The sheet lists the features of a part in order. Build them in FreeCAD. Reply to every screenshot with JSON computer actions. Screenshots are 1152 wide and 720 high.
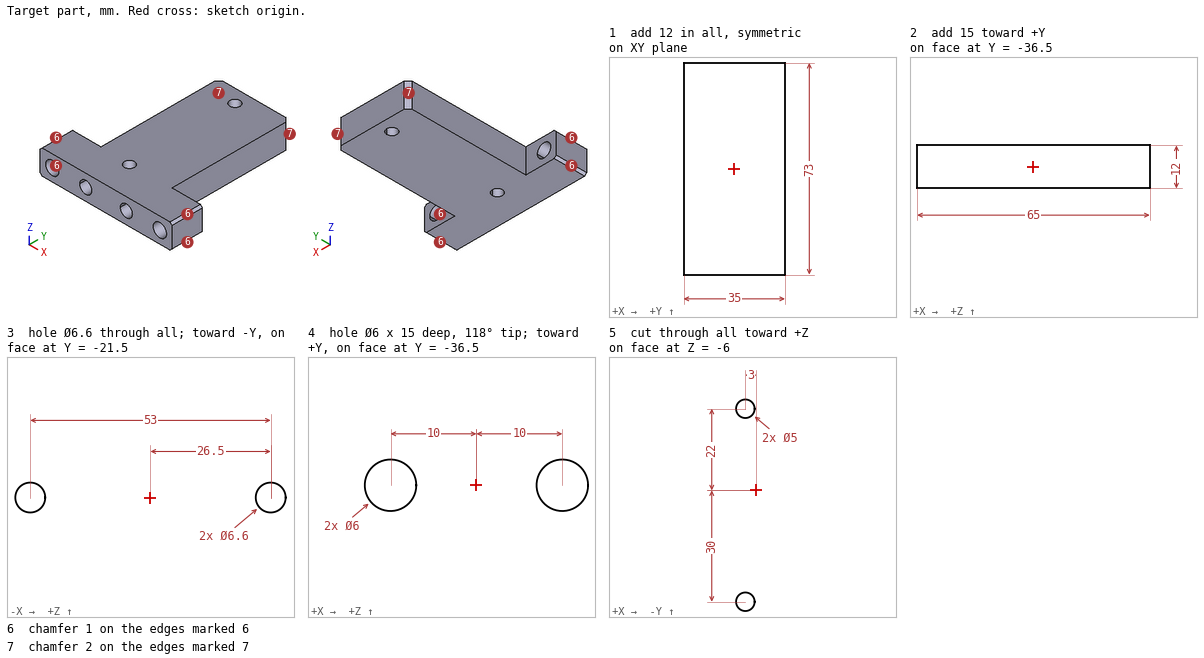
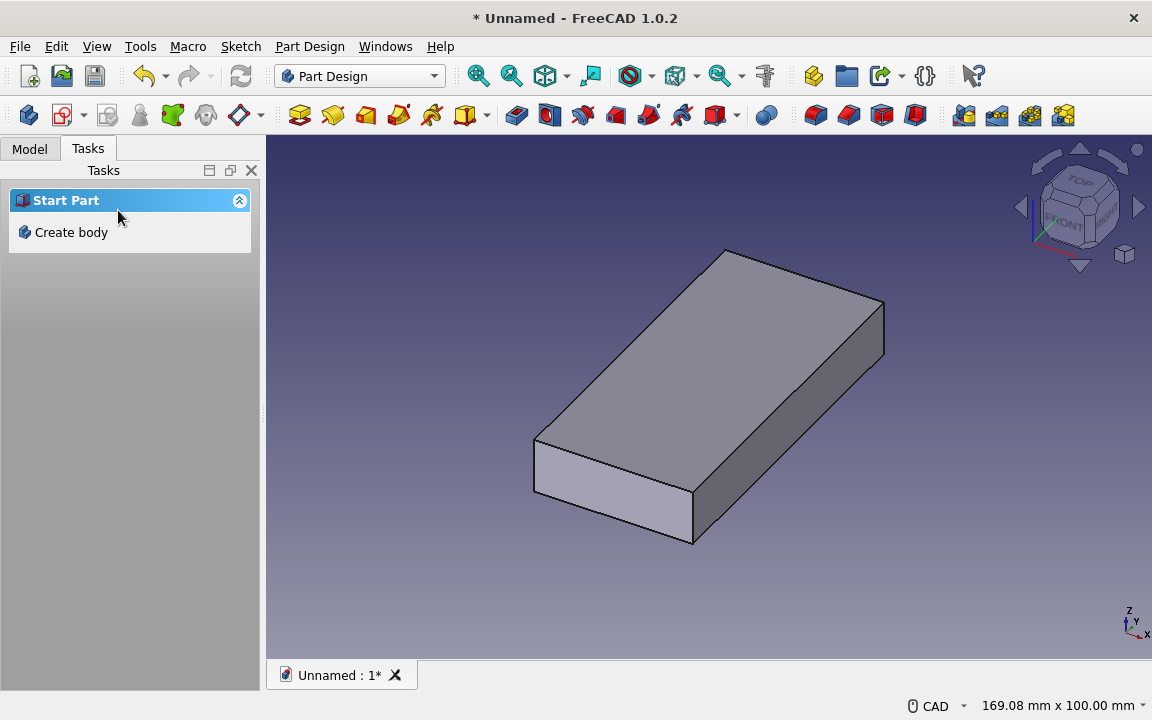
{"action": "left_click", "coordinate": [659, 506]}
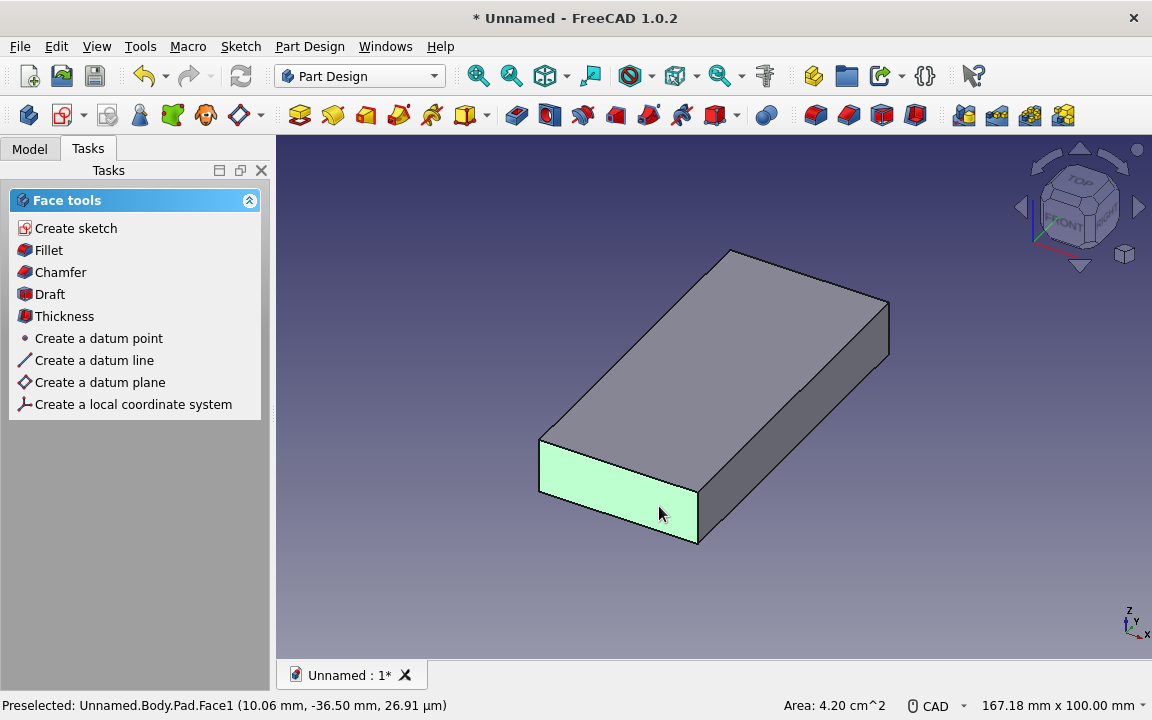
{"action": "left_click", "coordinate": [62, 116]}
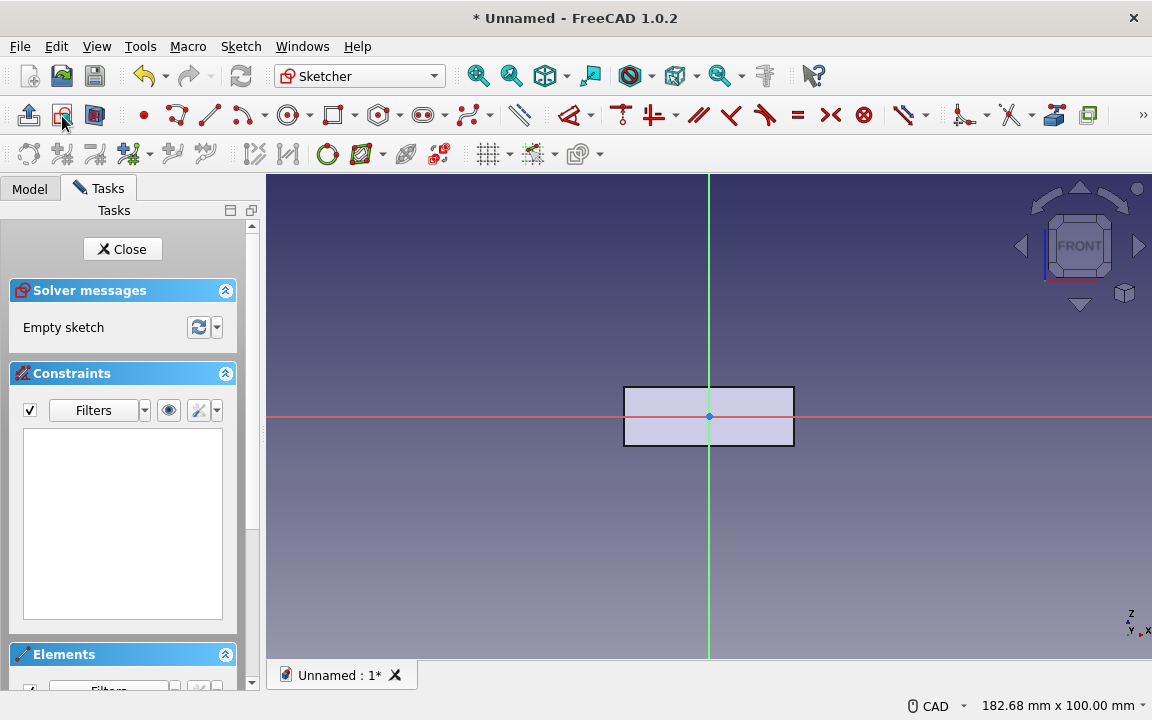
{"action": "scroll", "coordinate": [848, 416], "scroll_direction": "up", "scroll_amount": 2}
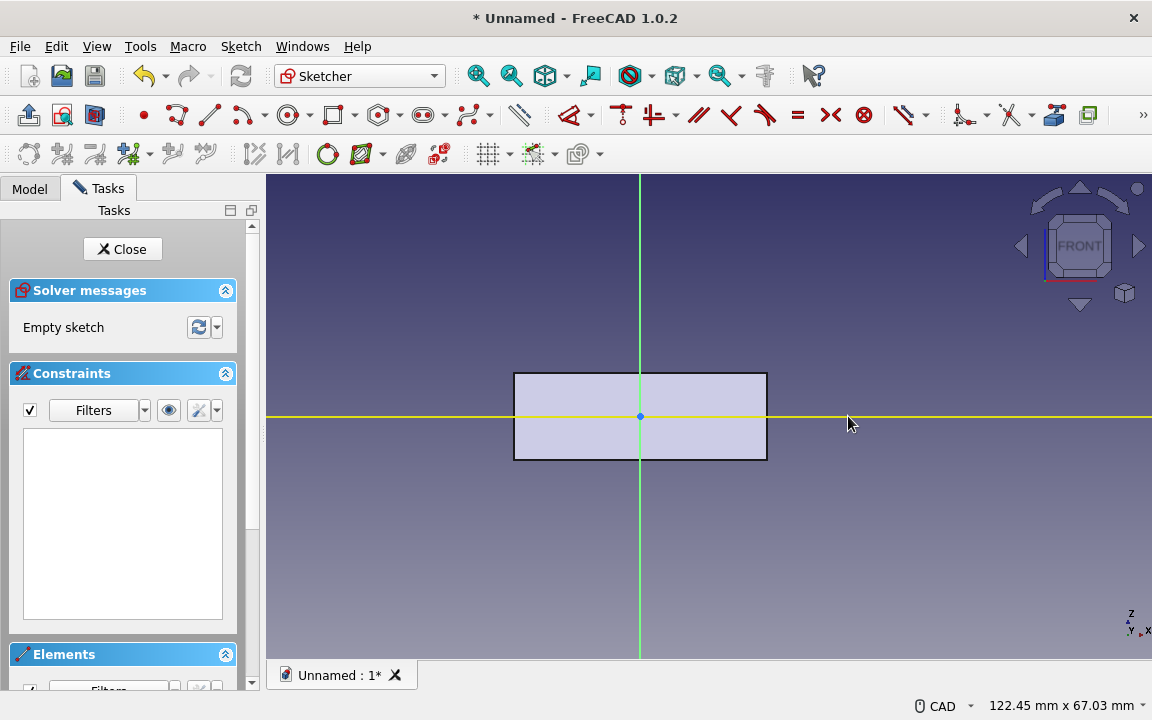
{"action": "key", "text": "g v"}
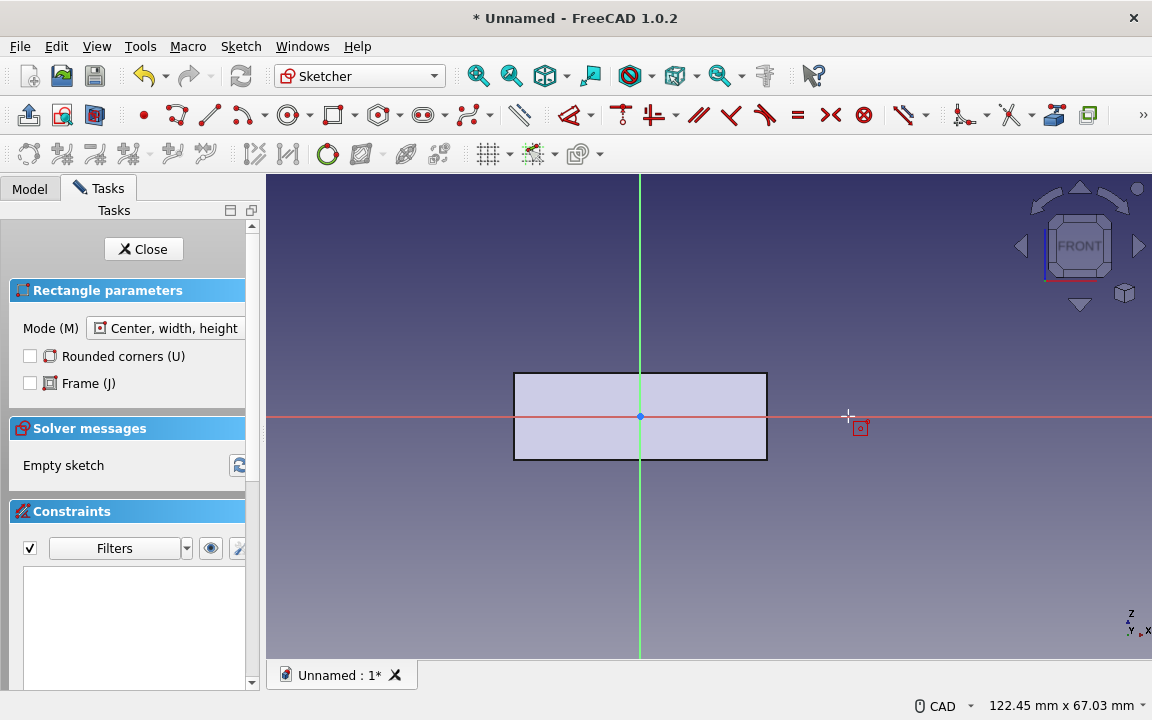
{"action": "left_click", "coordinate": [640, 416]}
{"action": "mouse_move", "coordinate": [875, 373]}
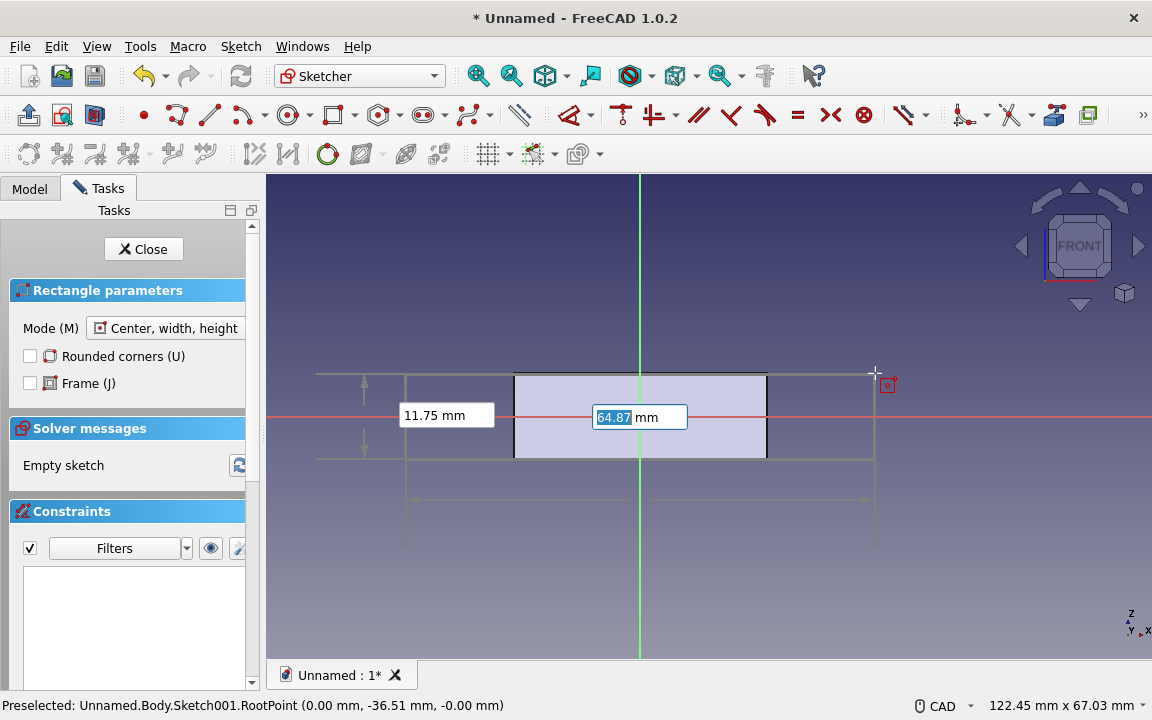
{"action": "type", "text": "65"}
{"action": "key", "text": "Tab"}
{"action": "type", "text": "12"}
{"action": "key", "text": "Return"}
{"action": "key", "text": "Escape"}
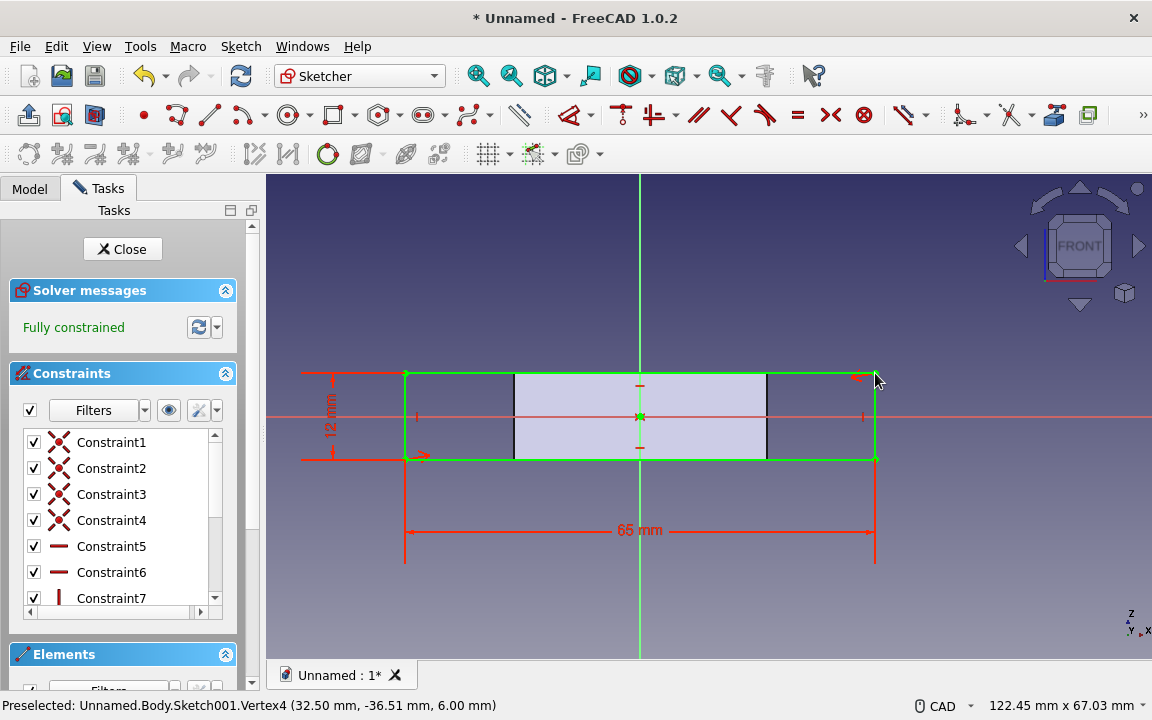
{"action": "left_click", "coordinate": [123, 249]}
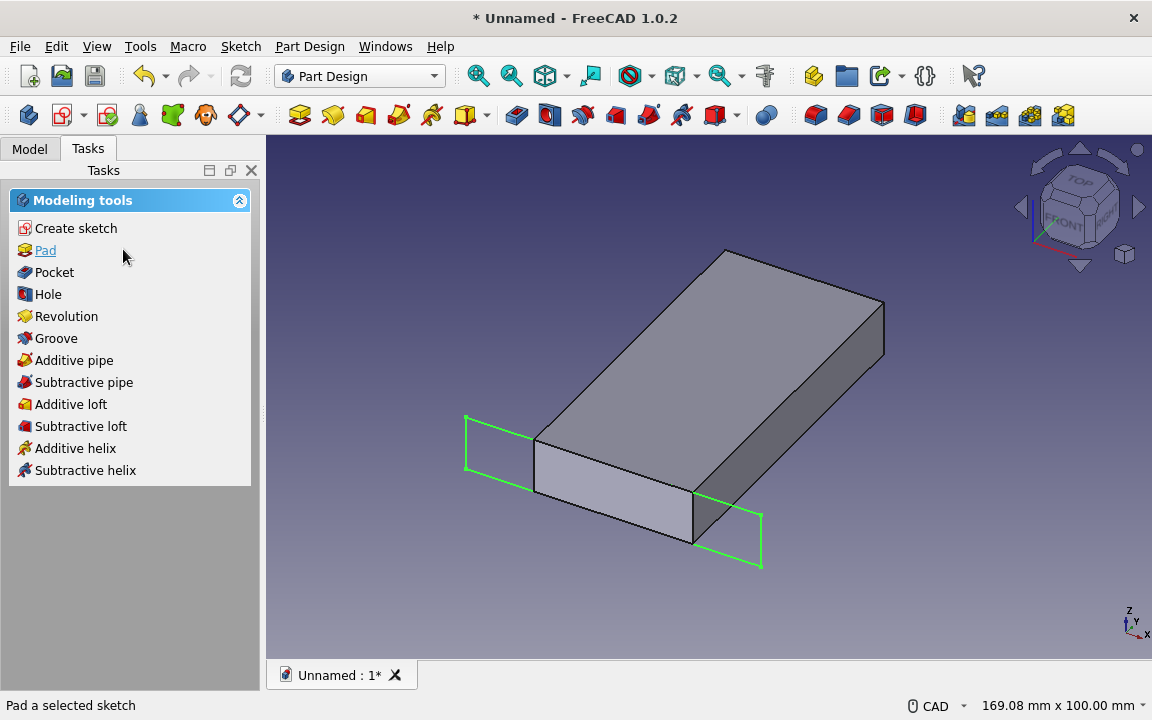
{"action": "left_click", "coordinate": [300, 116]}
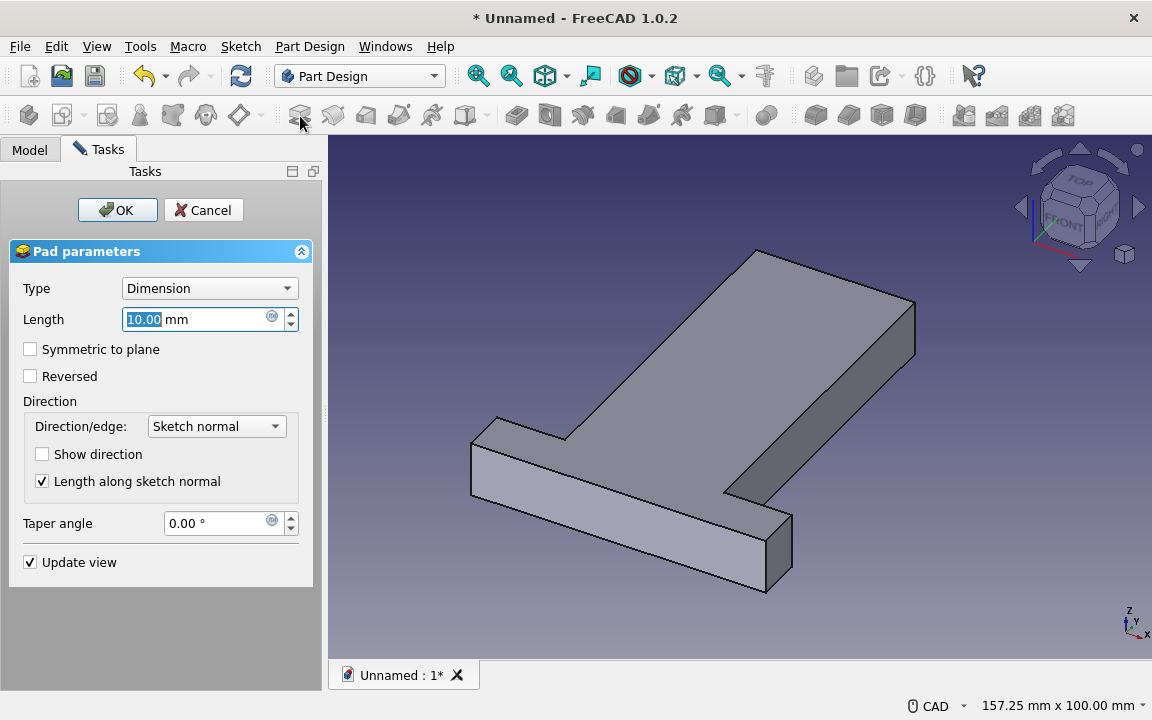
{"action": "type", "text": "15"}
{"action": "key", "text": "Tab"}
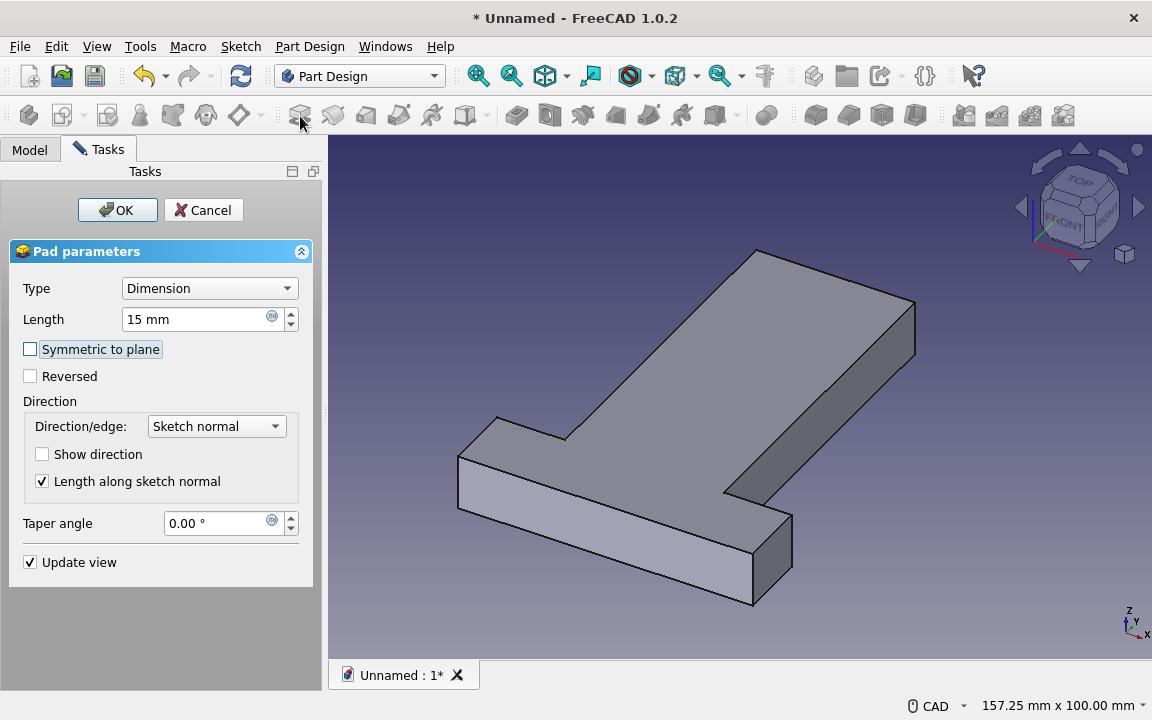
{"action": "left_click", "coordinate": [31, 376]}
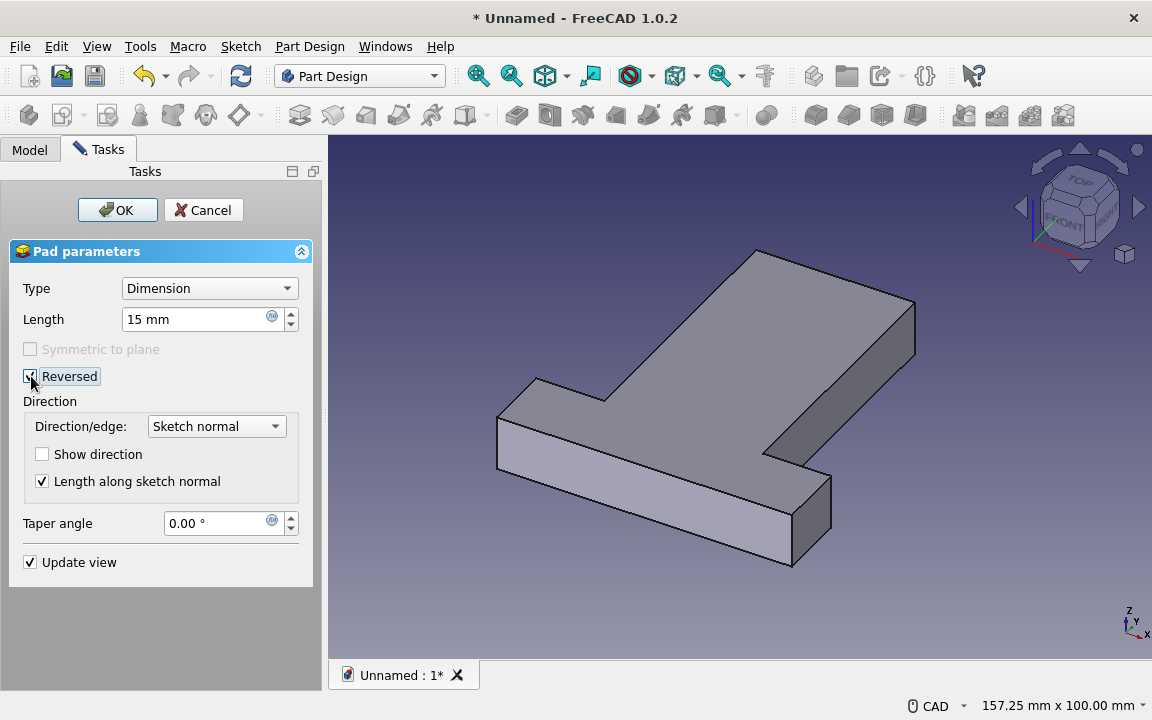
{"action": "left_click", "coordinate": [118, 210]}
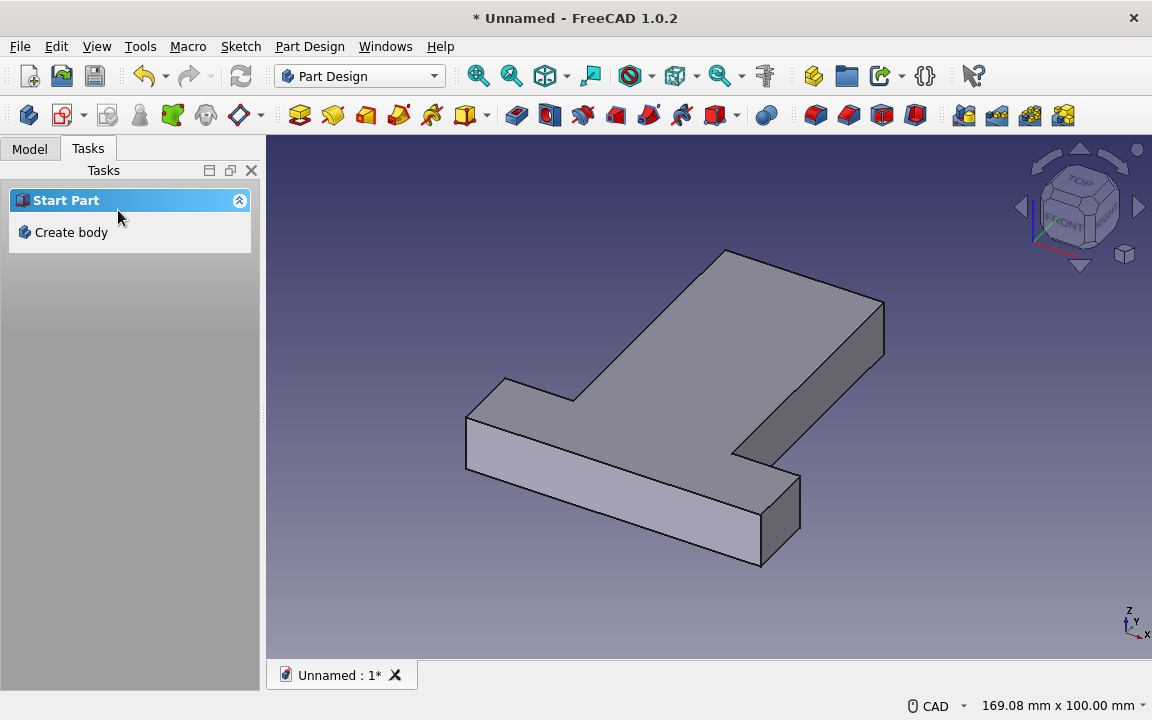
{"action": "key", "text": "4"}